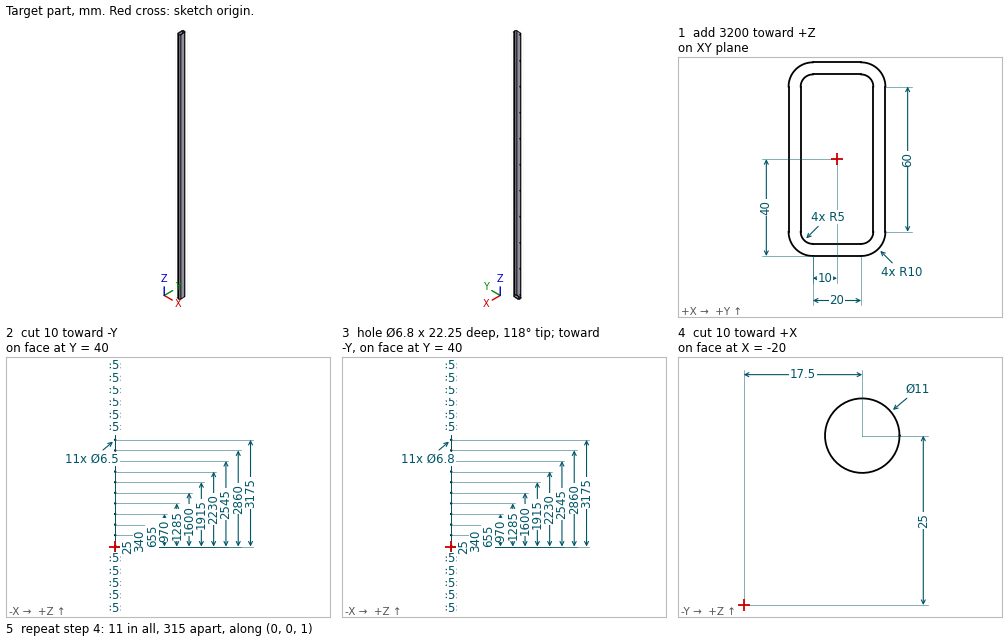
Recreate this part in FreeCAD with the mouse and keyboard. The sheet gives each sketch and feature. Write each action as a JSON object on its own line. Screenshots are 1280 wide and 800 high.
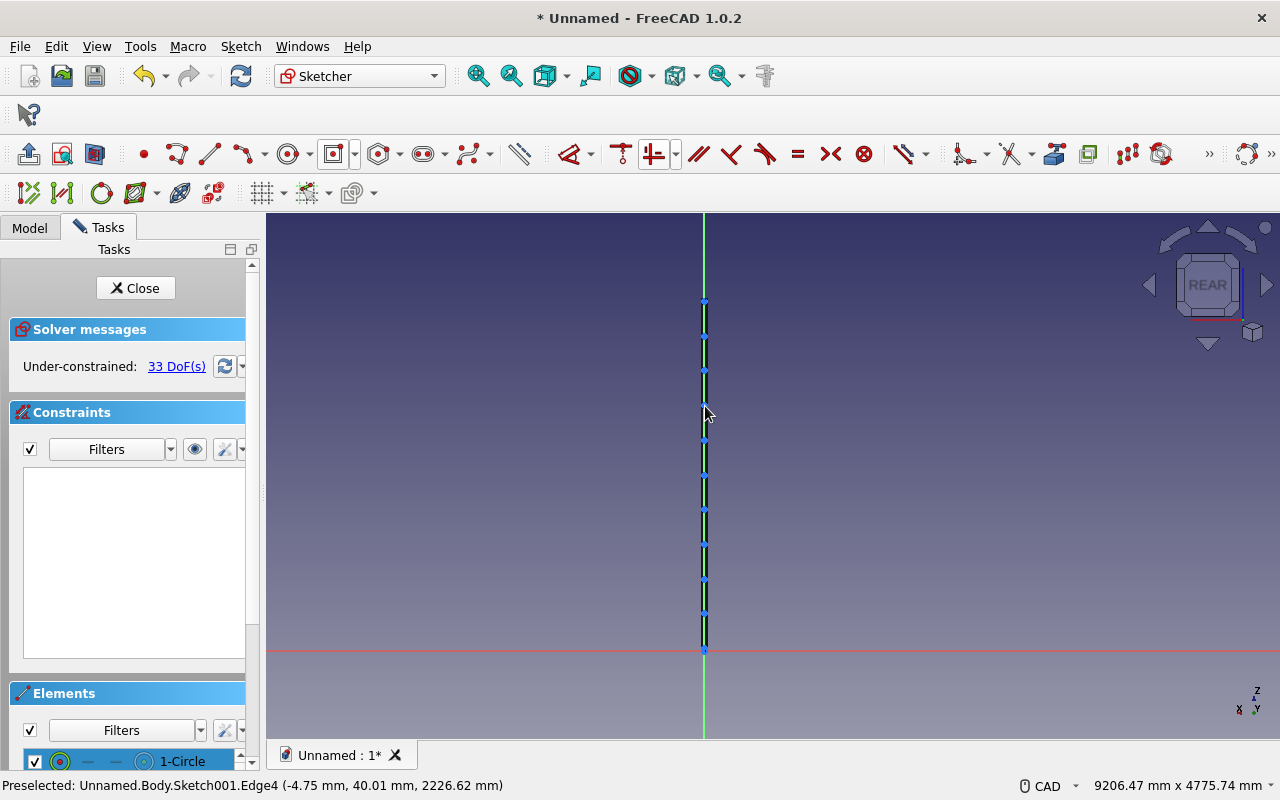
{"action": "scroll", "coordinate": [705, 440], "scroll_direction": "up", "scroll_amount": 14}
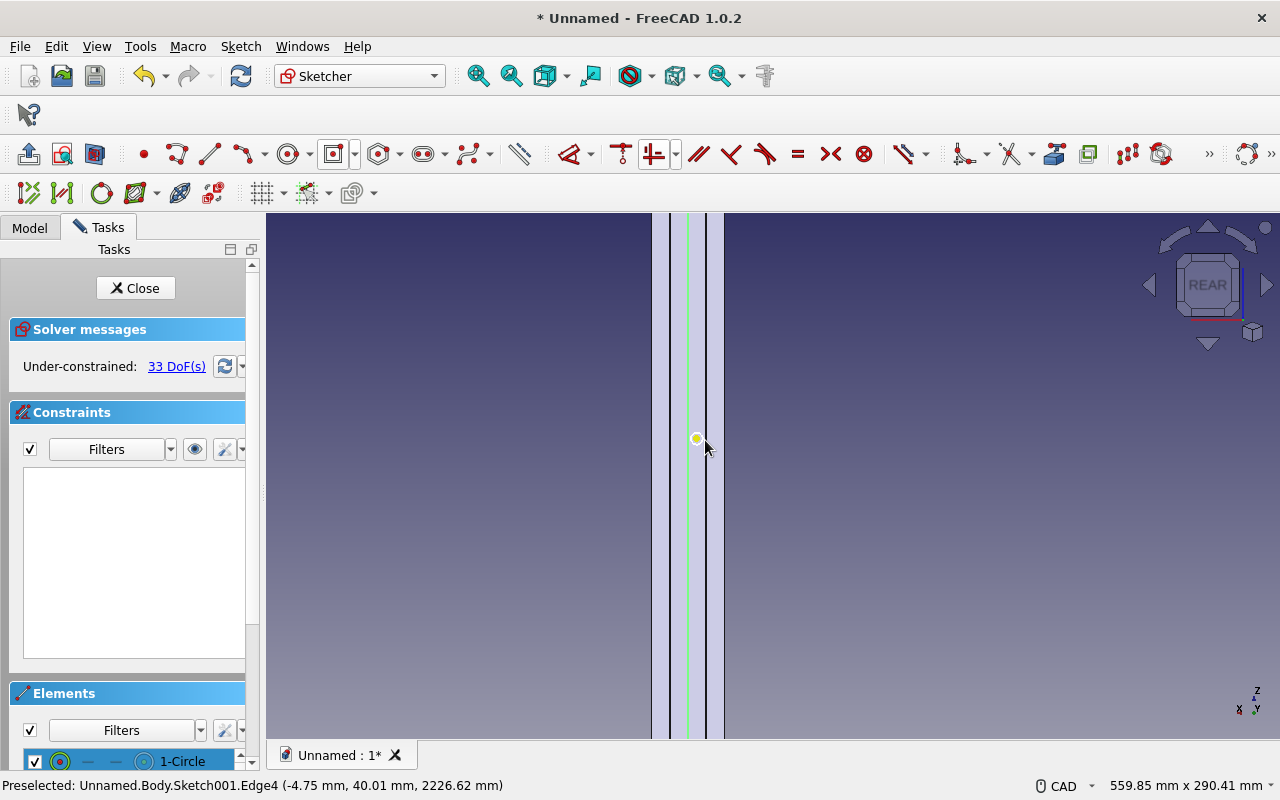
{"action": "left_click", "coordinate": [697, 445]}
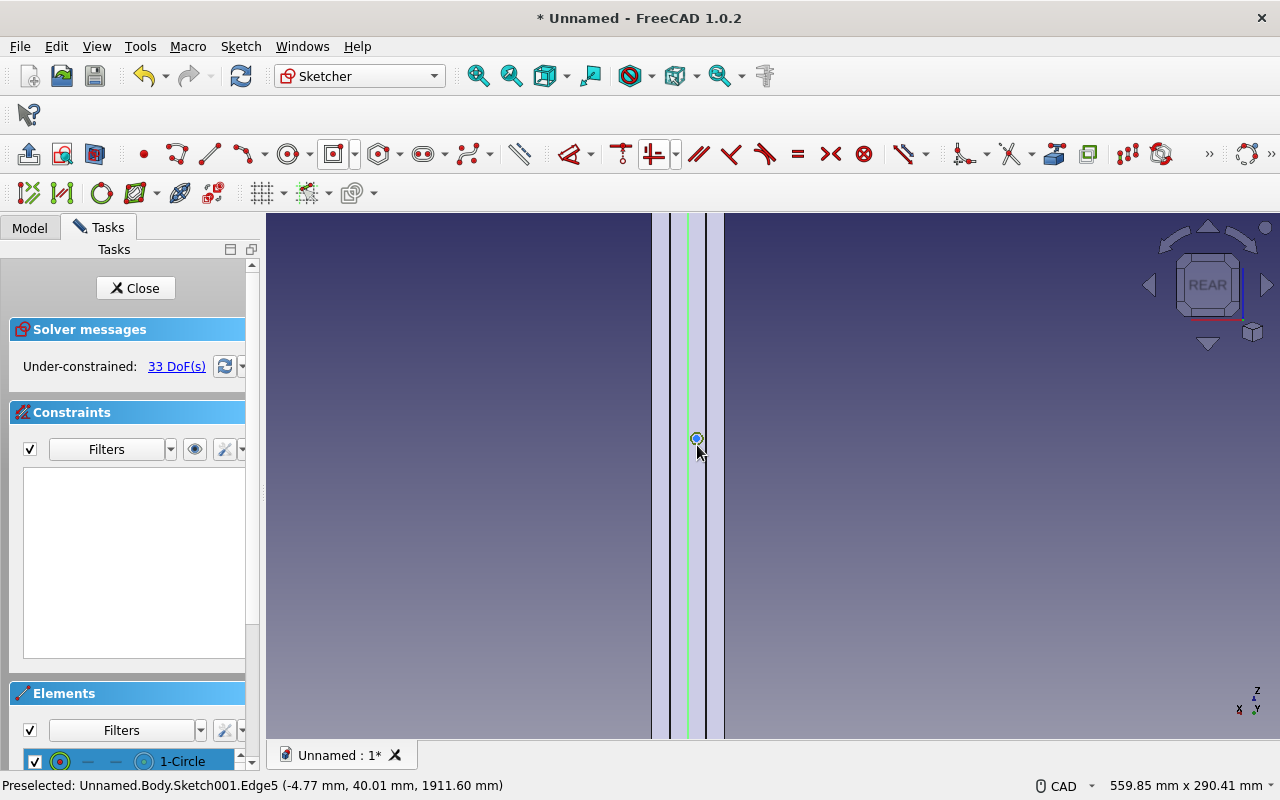
{"action": "scroll", "coordinate": [705, 440], "scroll_direction": "down", "scroll_amount": 14}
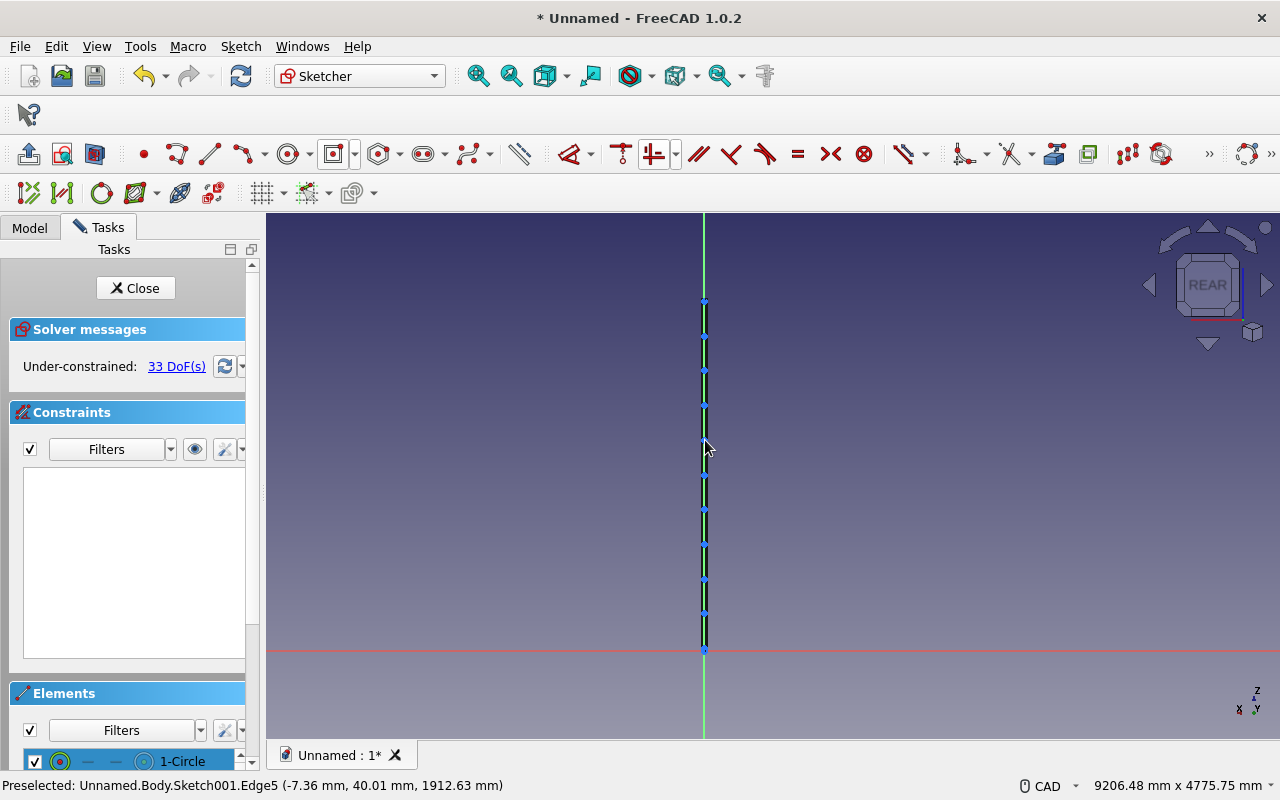
{"action": "scroll", "coordinate": [705, 475], "scroll_direction": "up", "scroll_amount": 14}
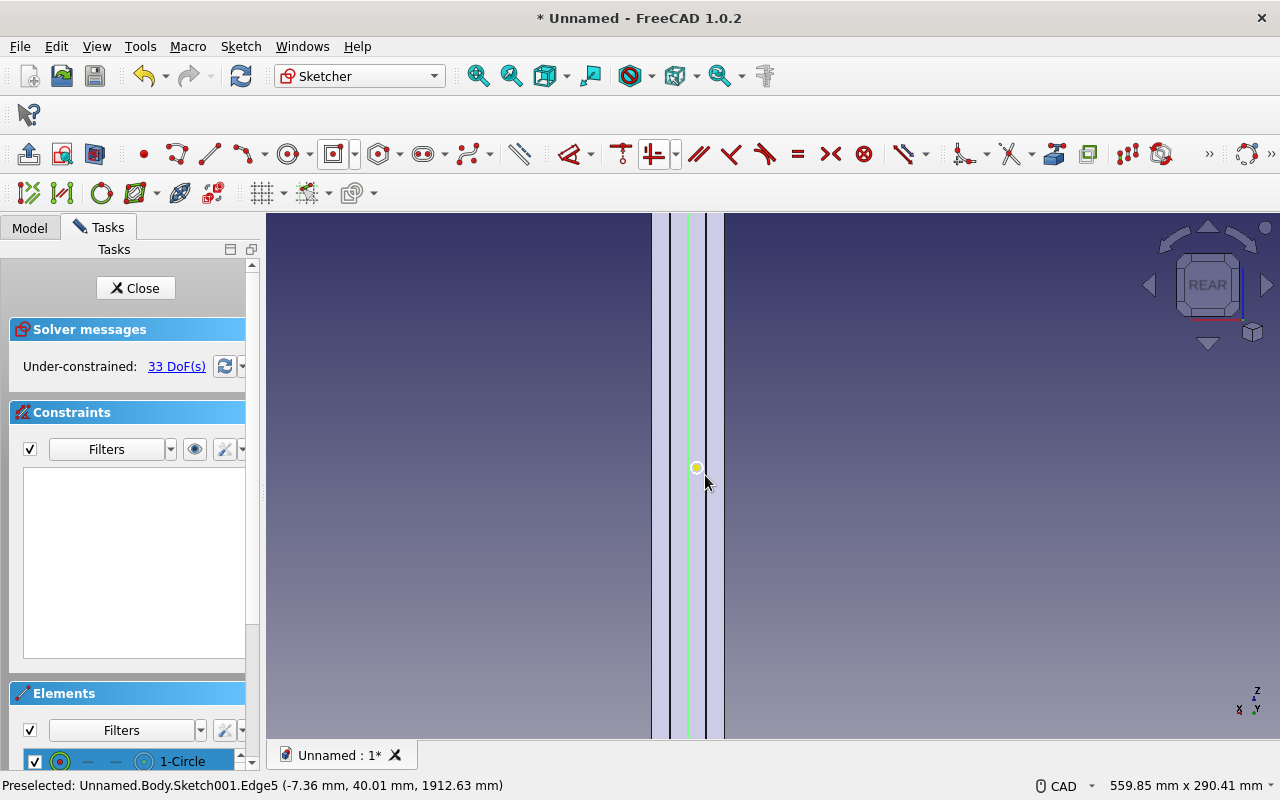
{"action": "left_click", "coordinate": [691, 467]}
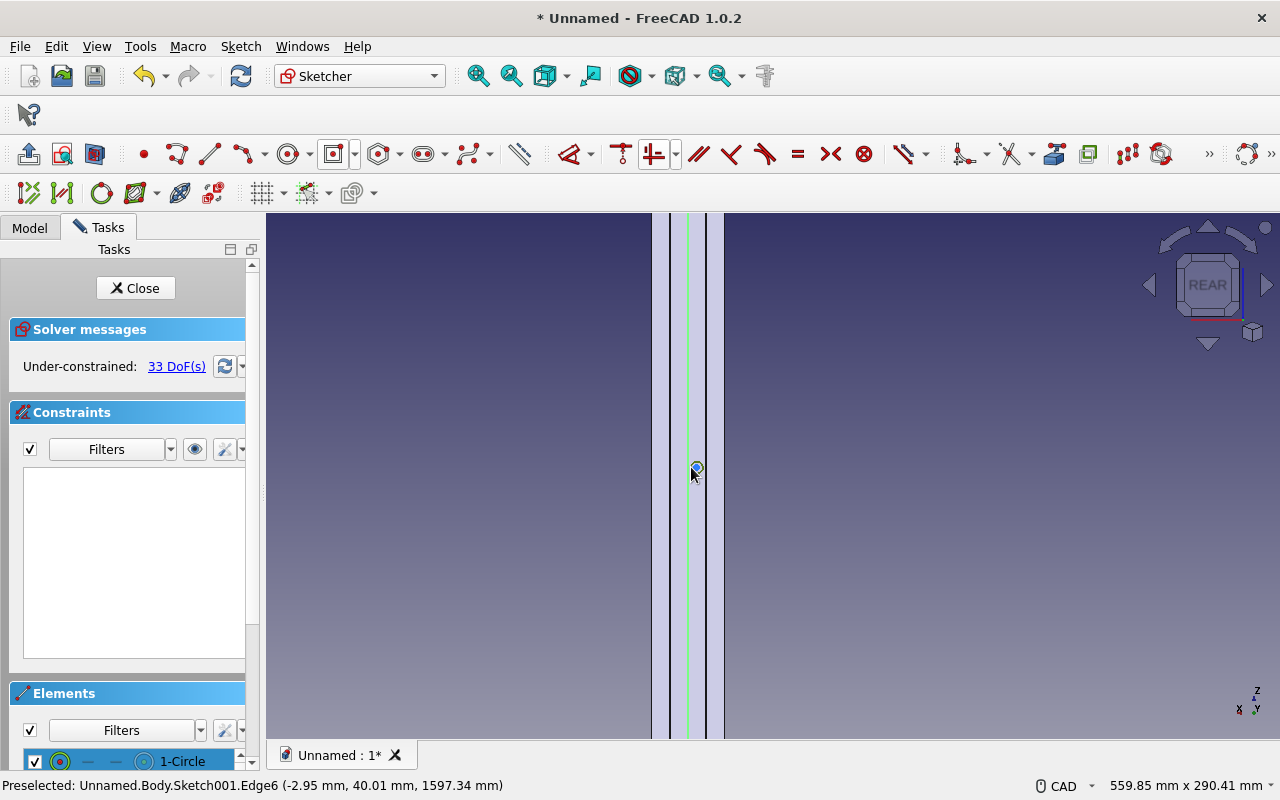
{"action": "scroll", "coordinate": [705, 475], "scroll_direction": "down", "scroll_amount": 14}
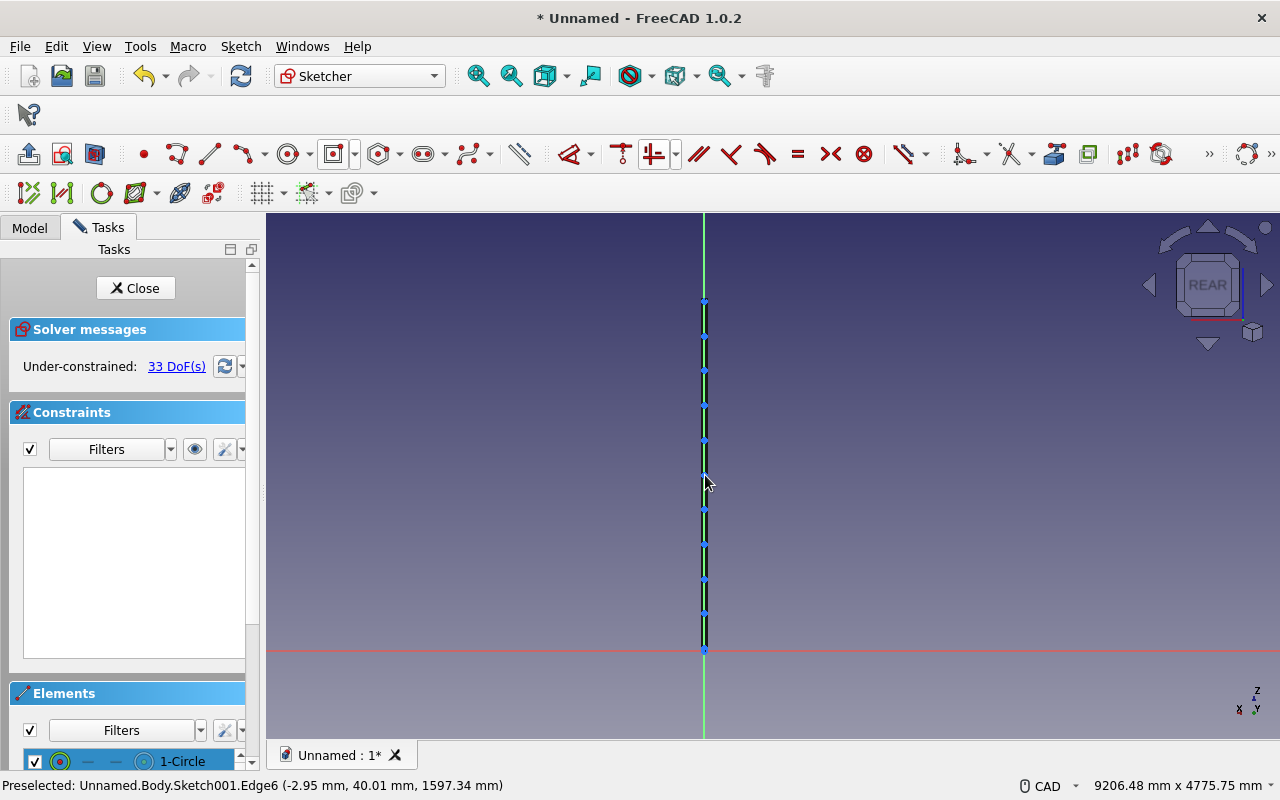
{"action": "scroll", "coordinate": [705, 509], "scroll_direction": "up", "scroll_amount": 14}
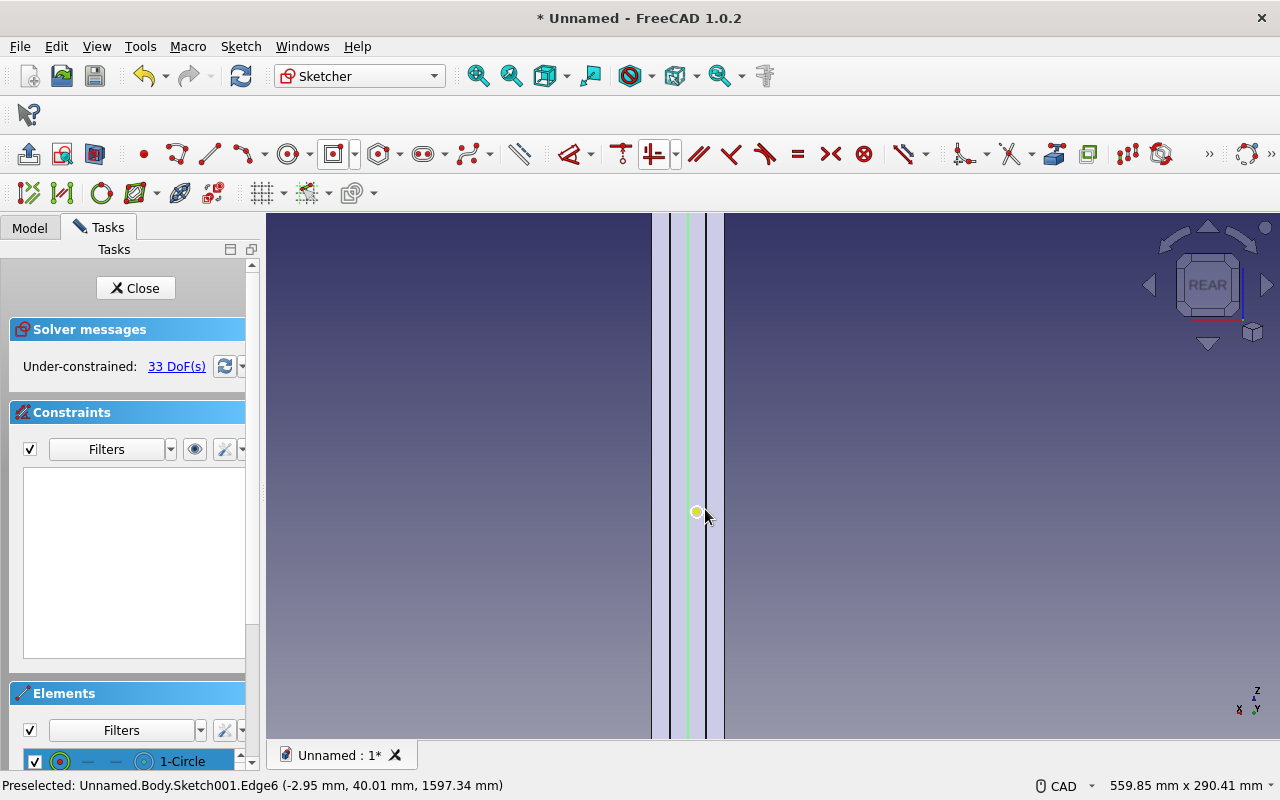
{"action": "left_click", "coordinate": [697, 518]}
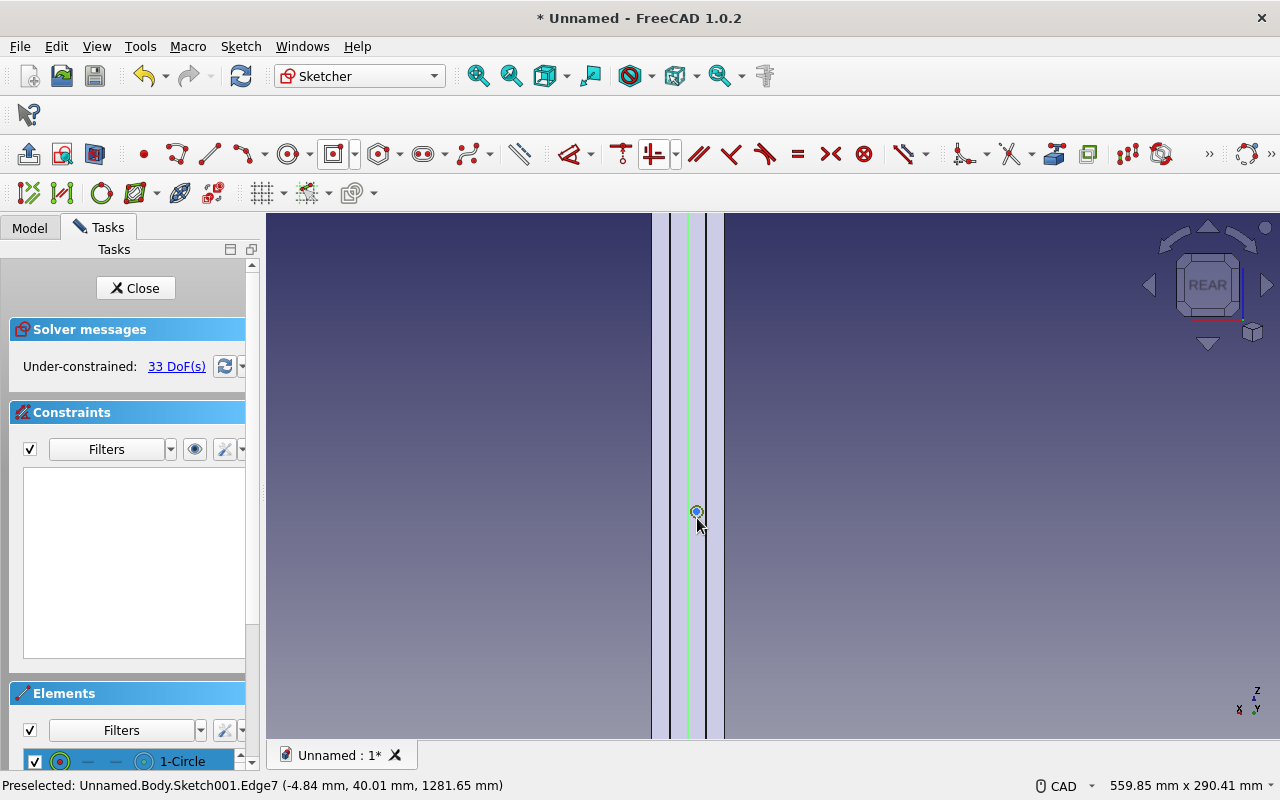
{"action": "scroll", "coordinate": [705, 509], "scroll_direction": "down", "scroll_amount": 14}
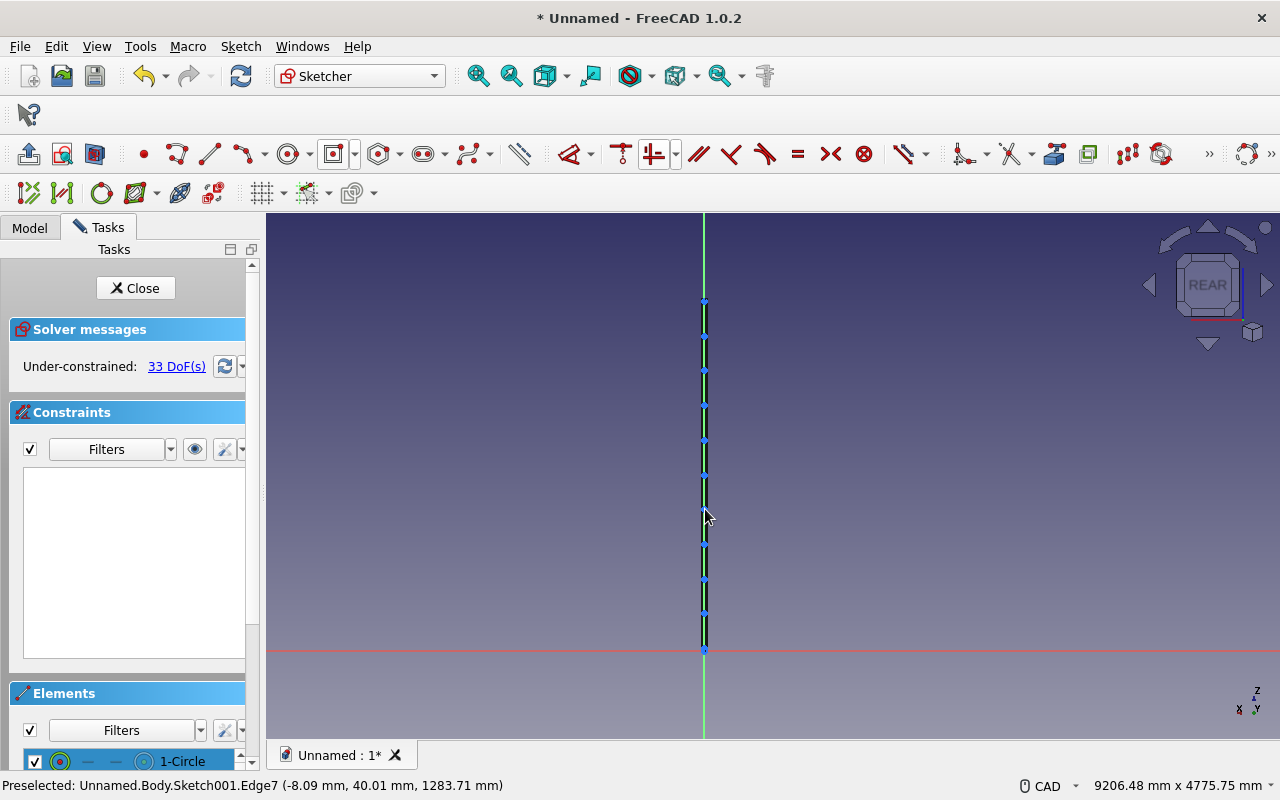
{"action": "scroll", "coordinate": [705, 545], "scroll_direction": "up", "scroll_amount": 14}